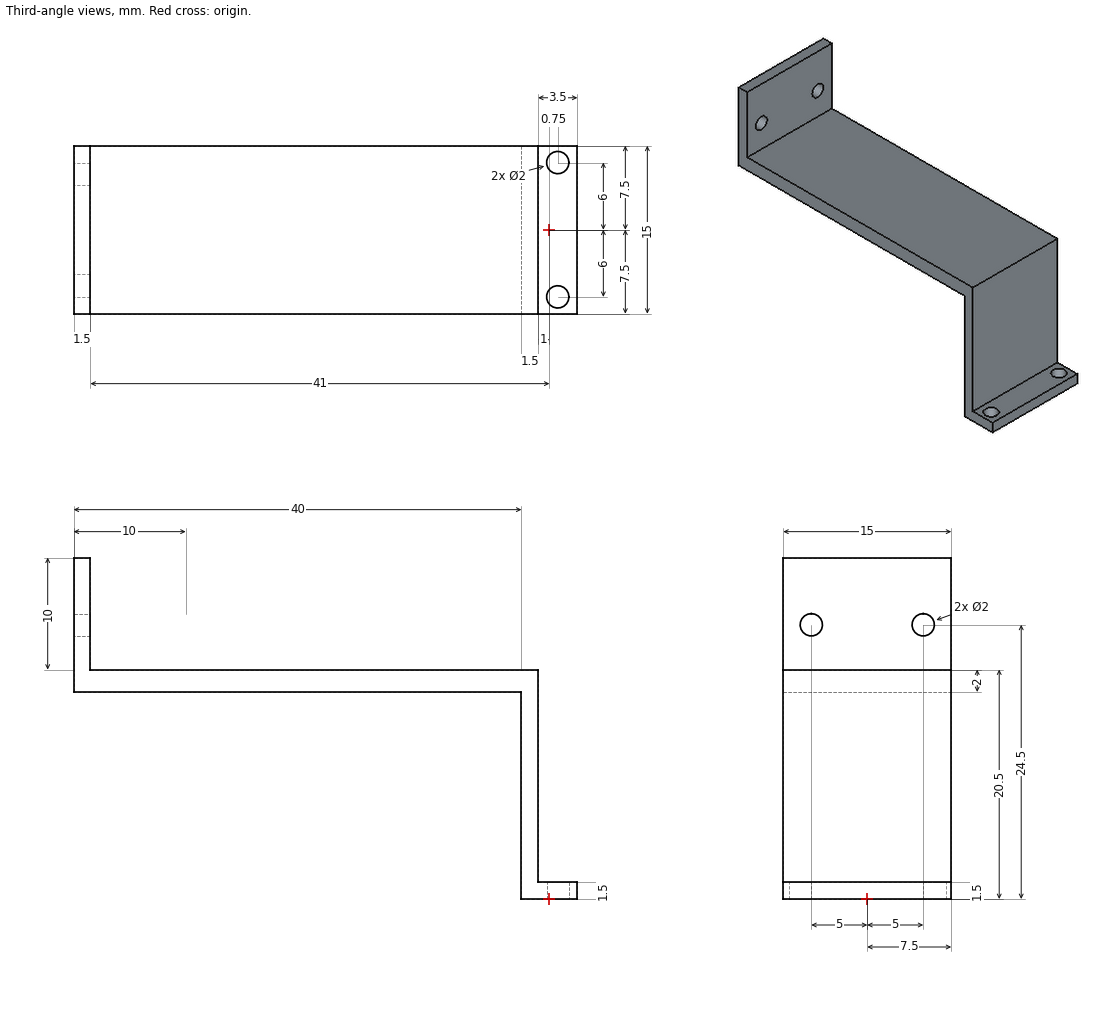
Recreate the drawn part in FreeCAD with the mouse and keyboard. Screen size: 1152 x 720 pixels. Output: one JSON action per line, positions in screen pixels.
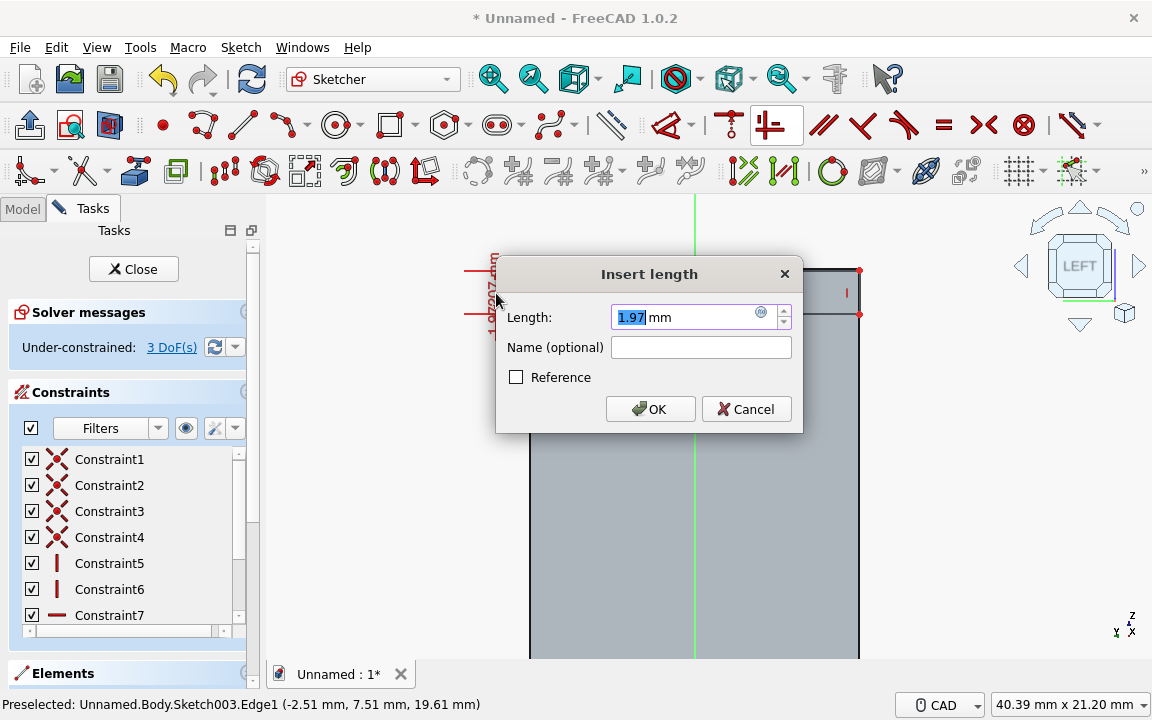
{"action": "type", "text": "2"}
{"action": "key", "text": "Return"}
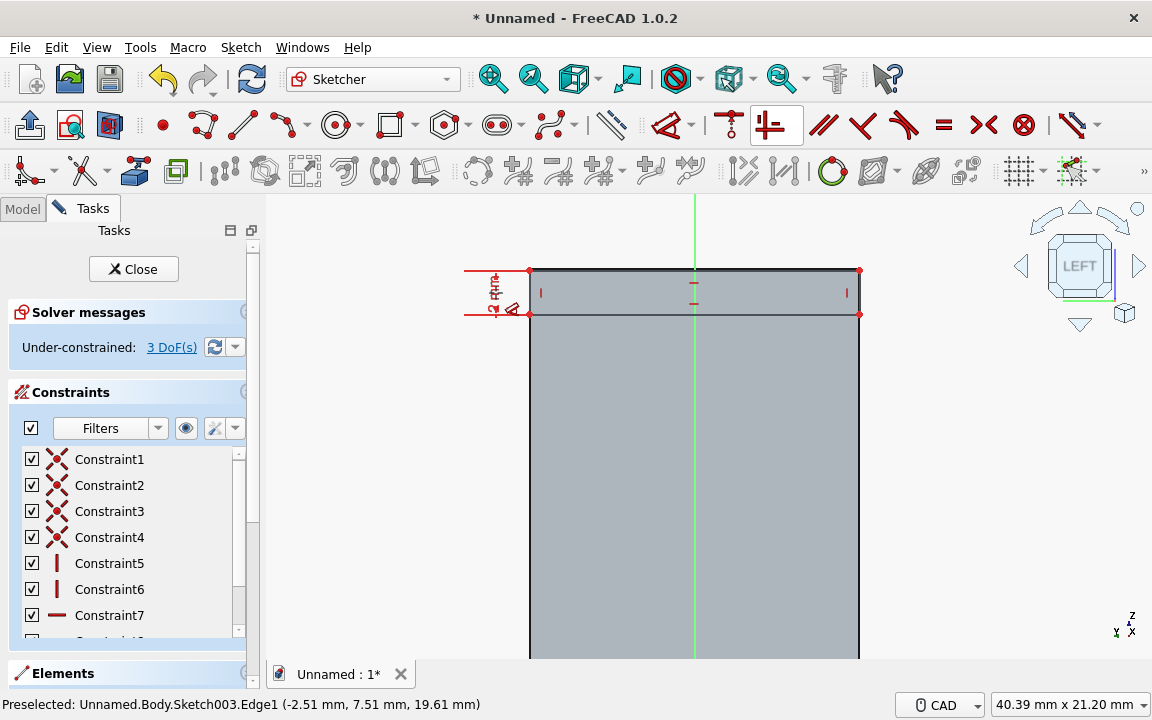
{"action": "left_click", "coordinate": [629, 315]}
{"action": "left_click", "coordinate": [619, 349]}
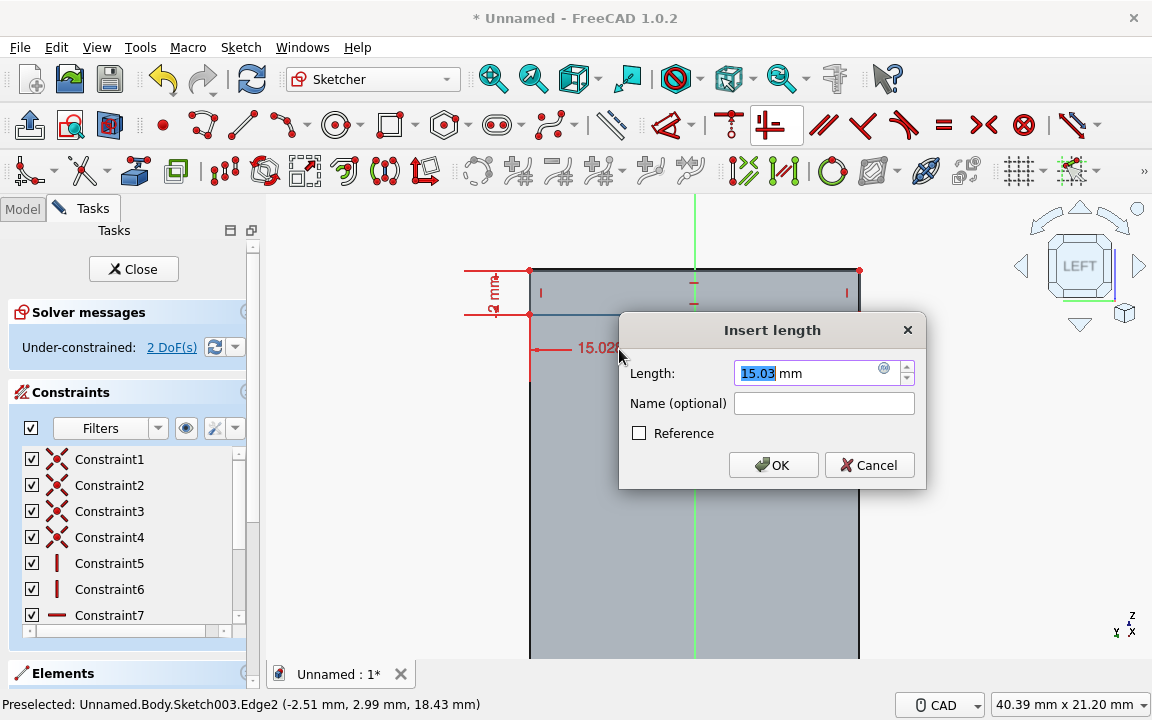
{"action": "type", "text": "15"}
{"action": "key", "text": "Return"}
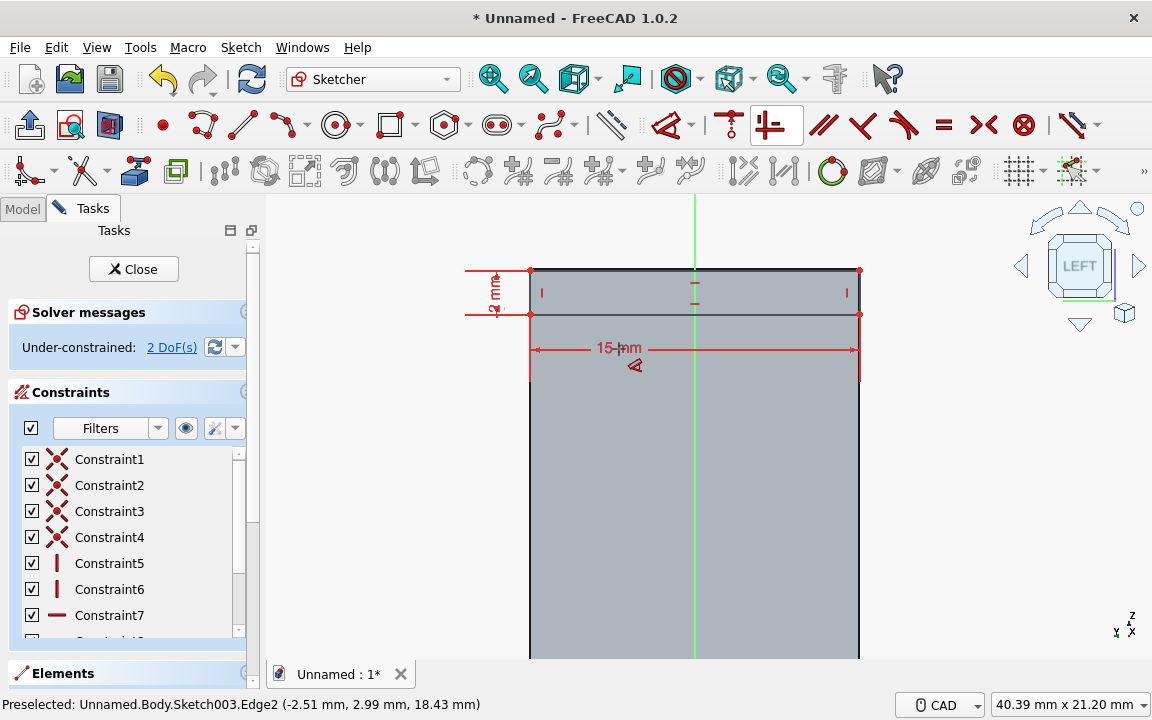
{"action": "left_click", "coordinate": [530, 271]}
{"action": "left_click", "coordinate": [613, 237]}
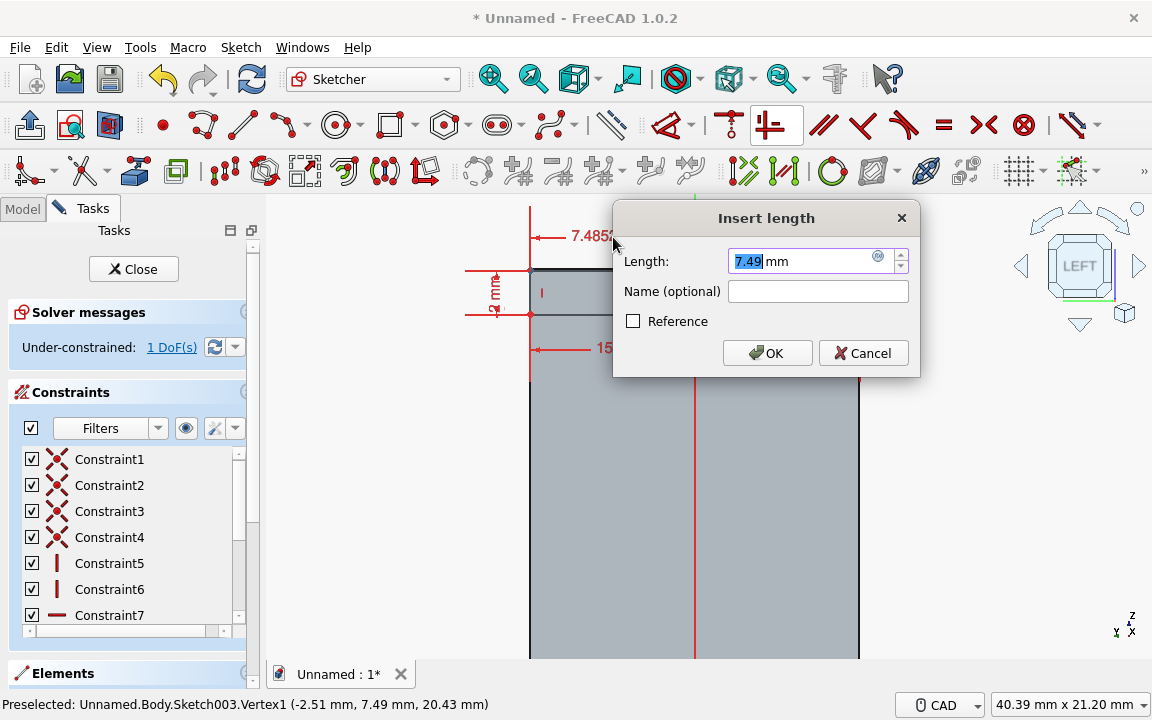
{"action": "type", "text": "7.5"}
{"action": "key", "text": "Return"}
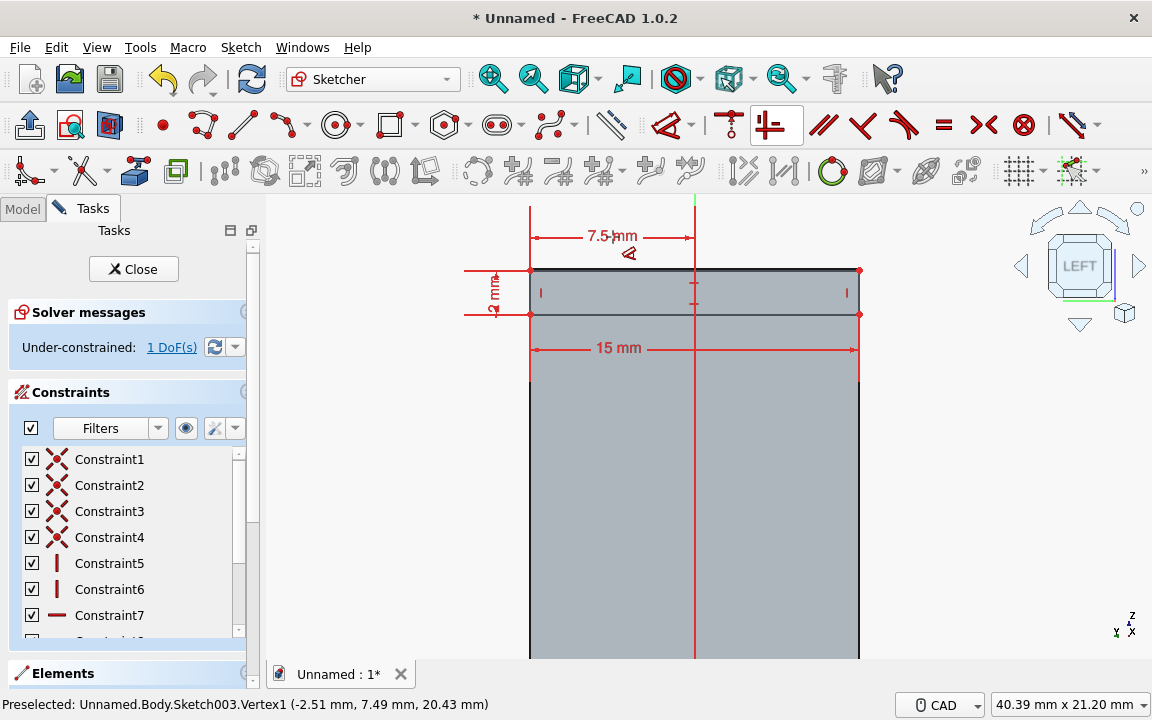
{"action": "left_click", "coordinate": [530, 271]}
{"action": "left_click", "coordinate": [496, 451]}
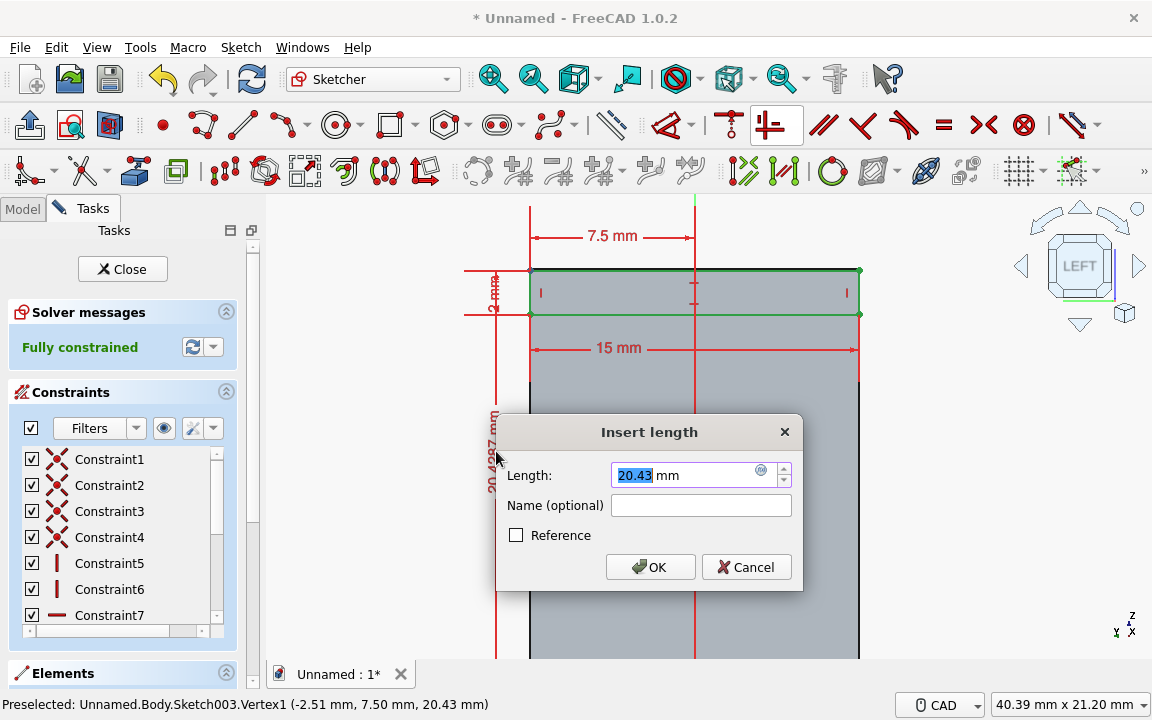
{"action": "type", "text": "20.5"}
{"action": "key", "text": "Return"}
{"action": "key", "text": "Escape"}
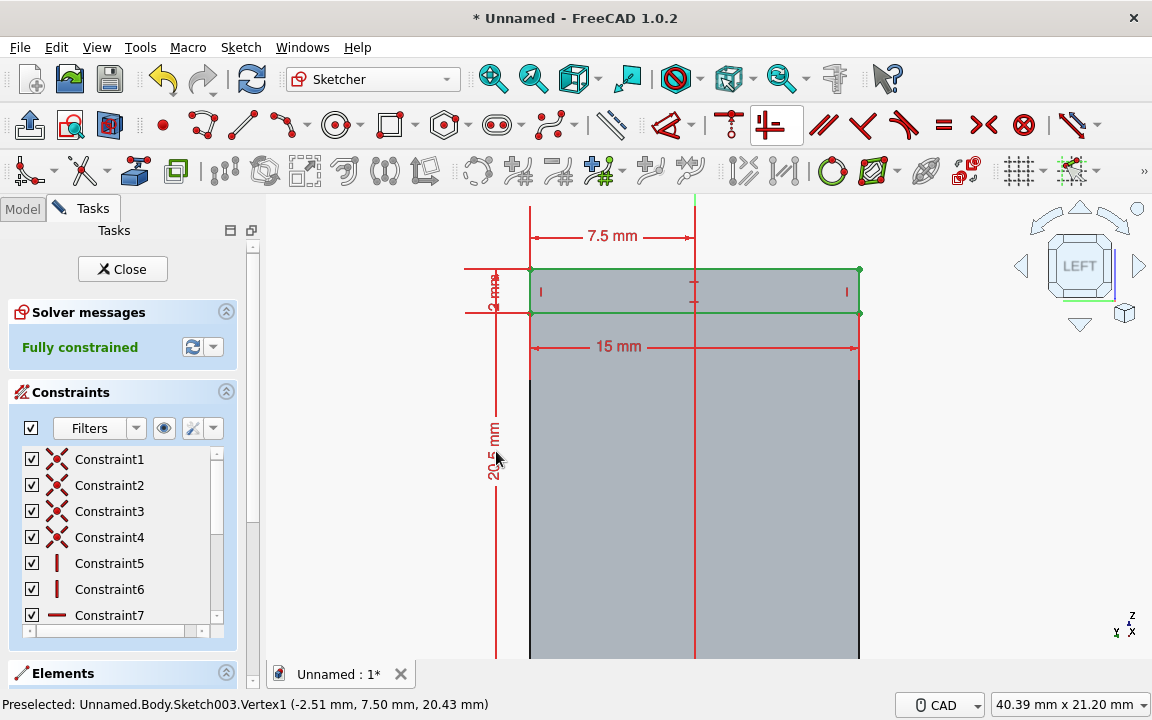
{"action": "left_click", "coordinate": [123, 269]}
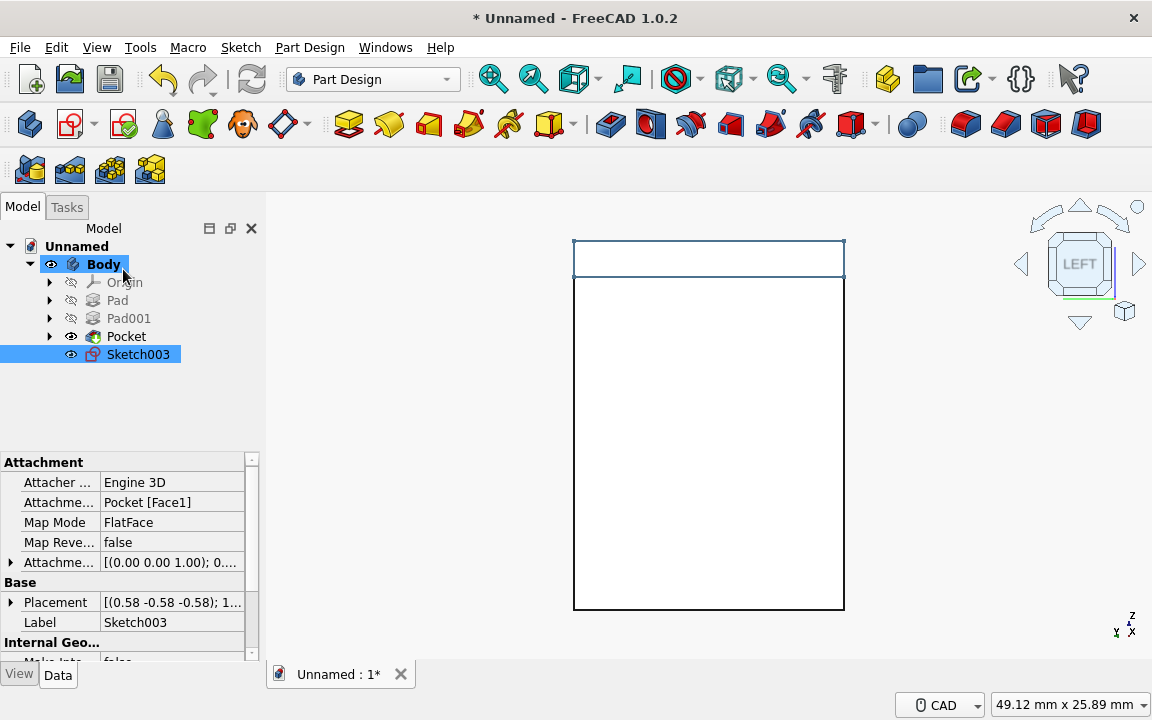
{"action": "left_click", "coordinate": [350, 124]}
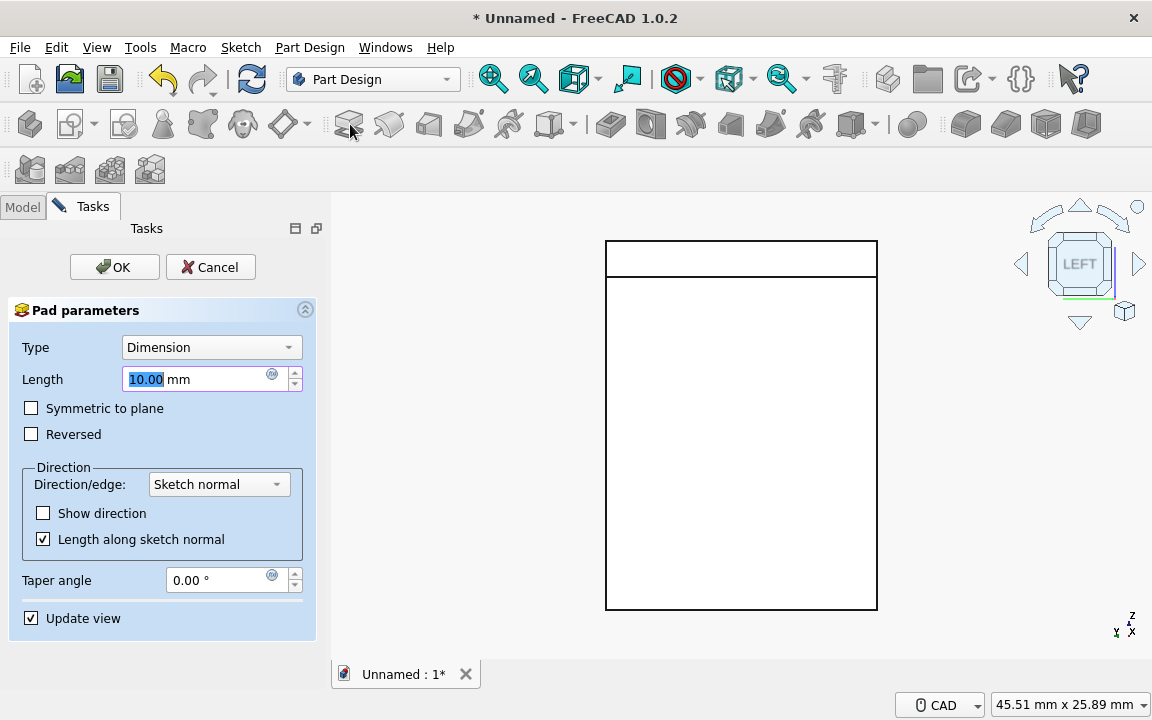
{"action": "type", "text": "40"}
{"action": "key", "text": "Tab"}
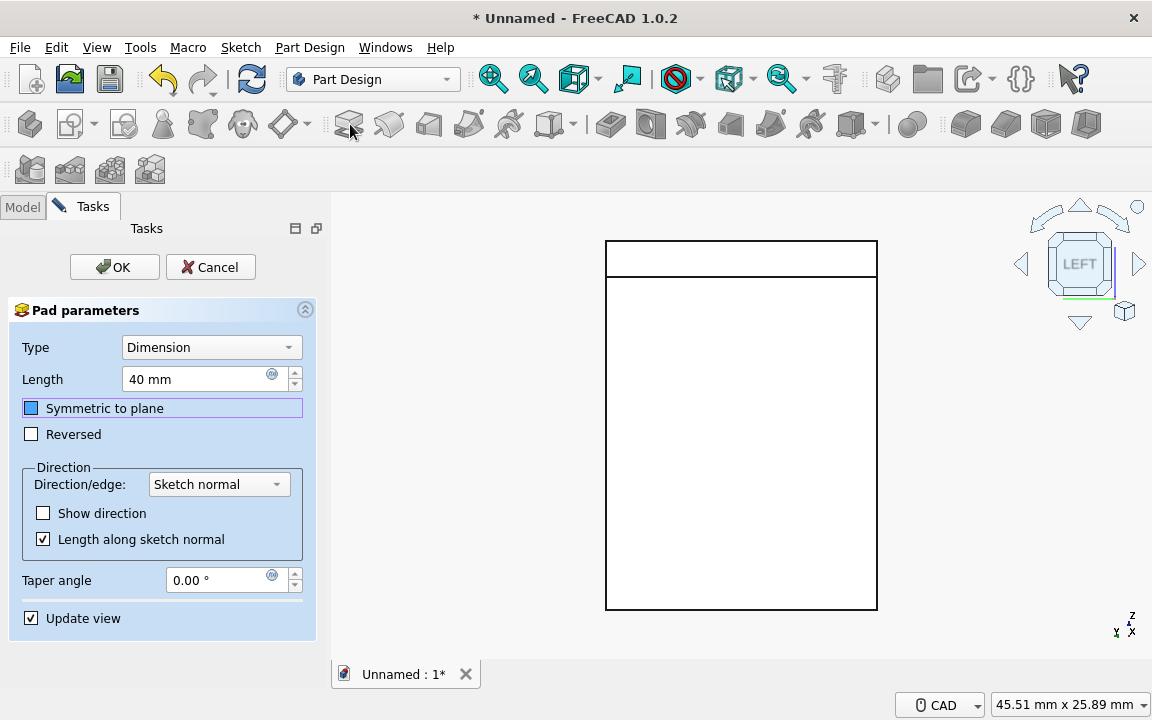
{"action": "left_click", "coordinate": [115, 267]}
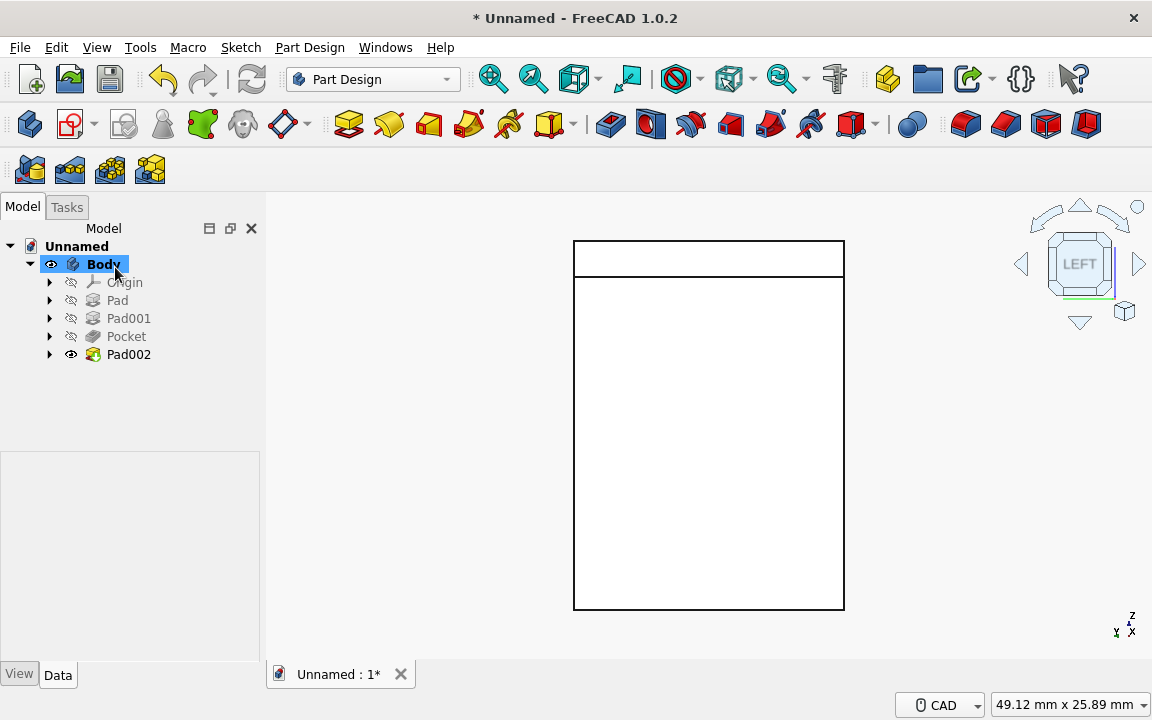
{"action": "key", "text": "0"}